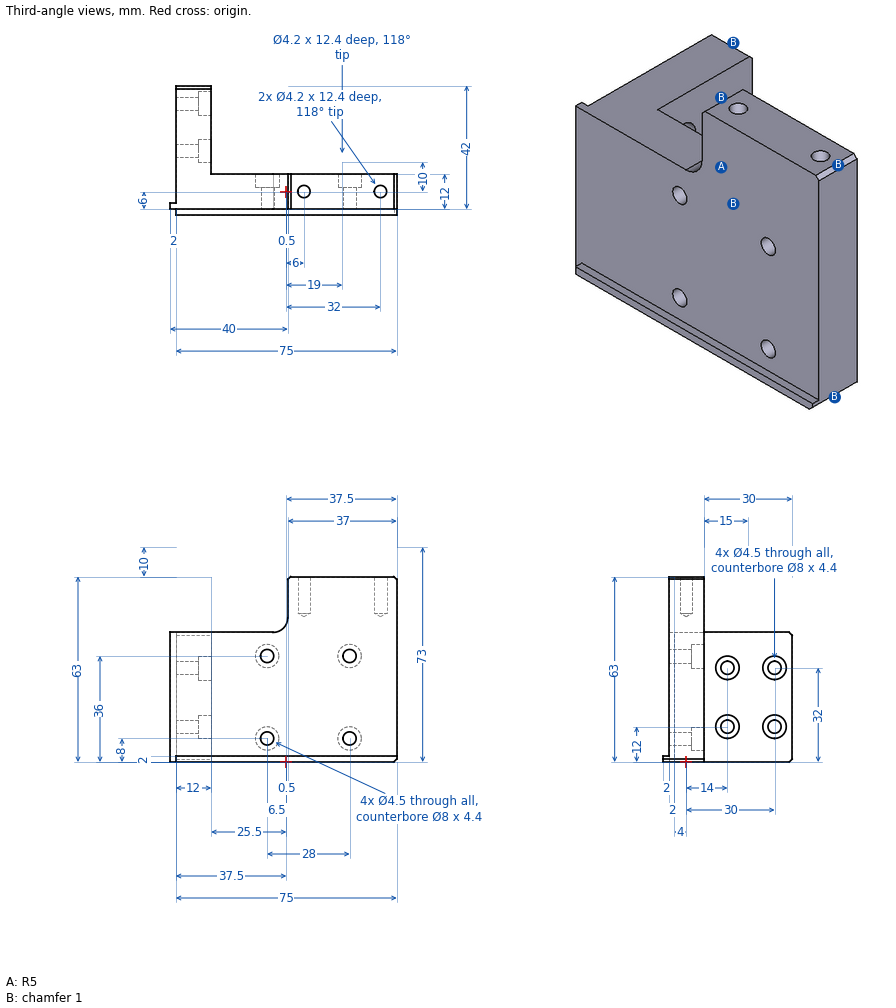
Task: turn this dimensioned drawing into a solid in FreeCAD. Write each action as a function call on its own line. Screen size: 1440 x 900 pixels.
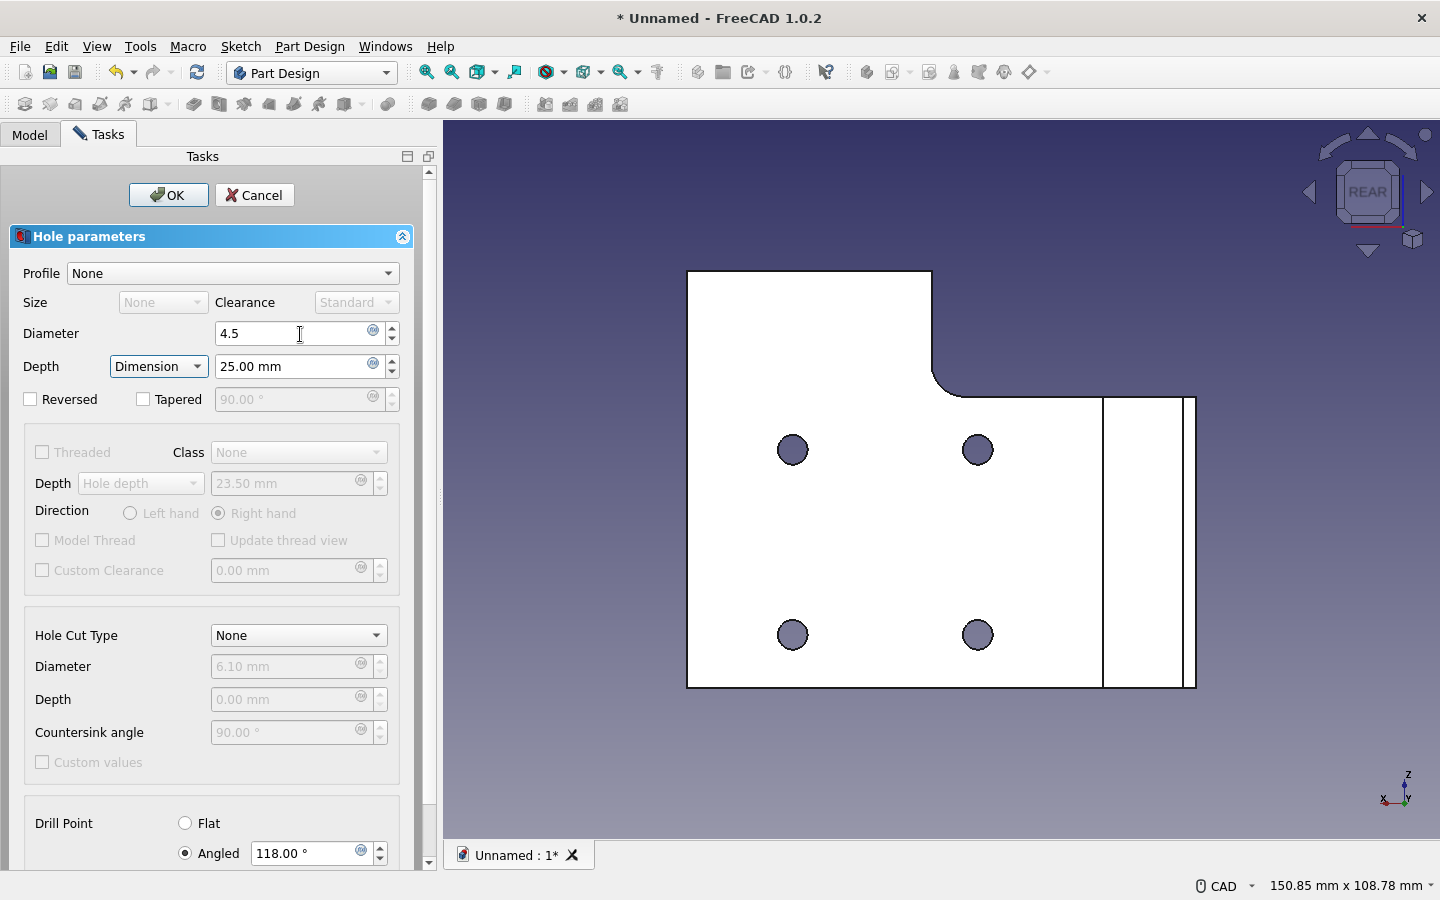
click(160, 366)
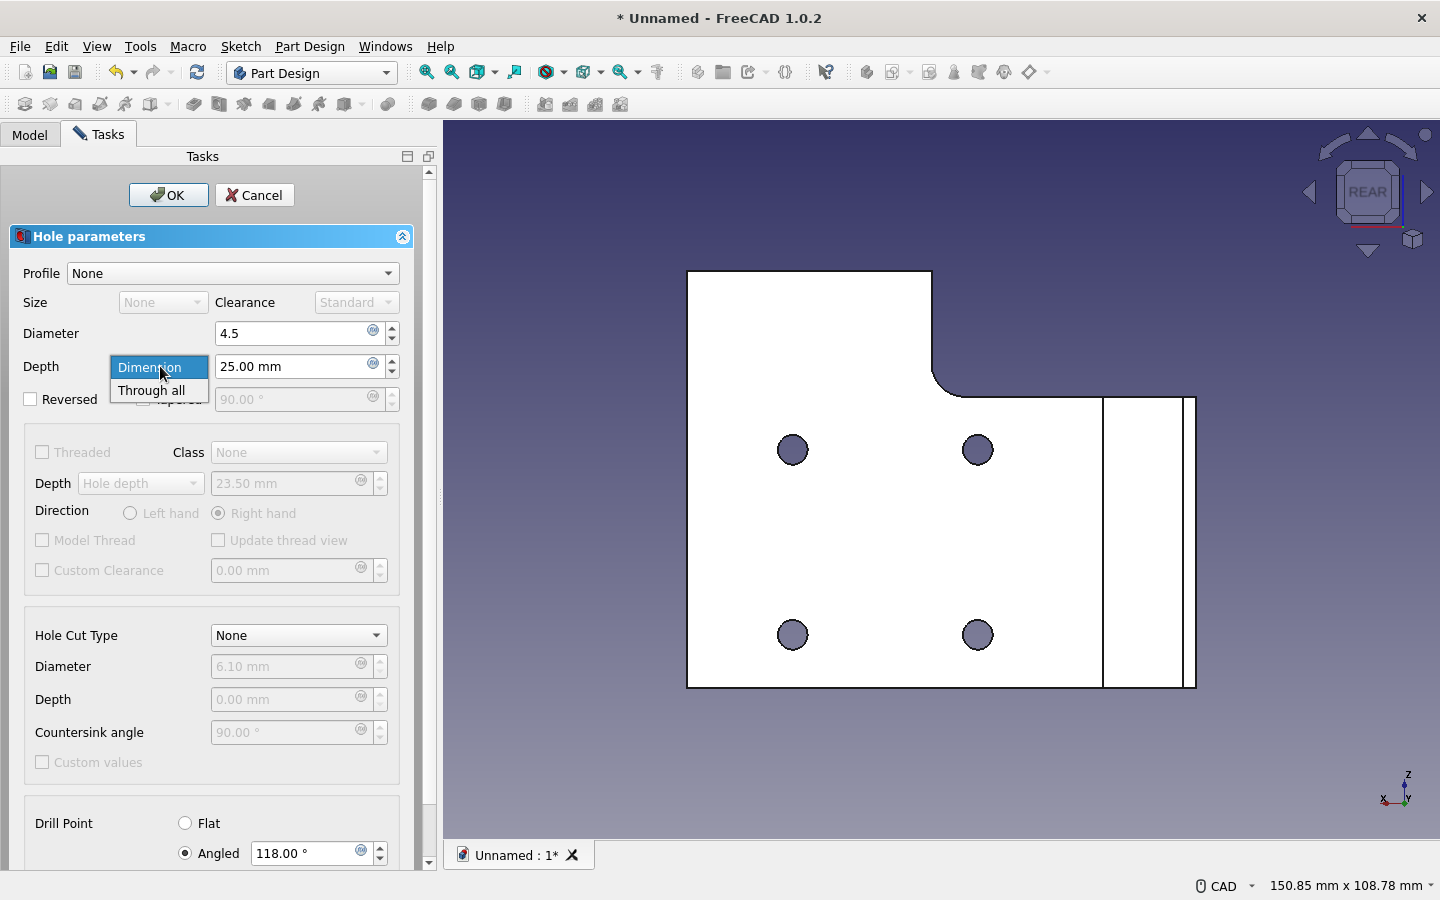
click(158, 390)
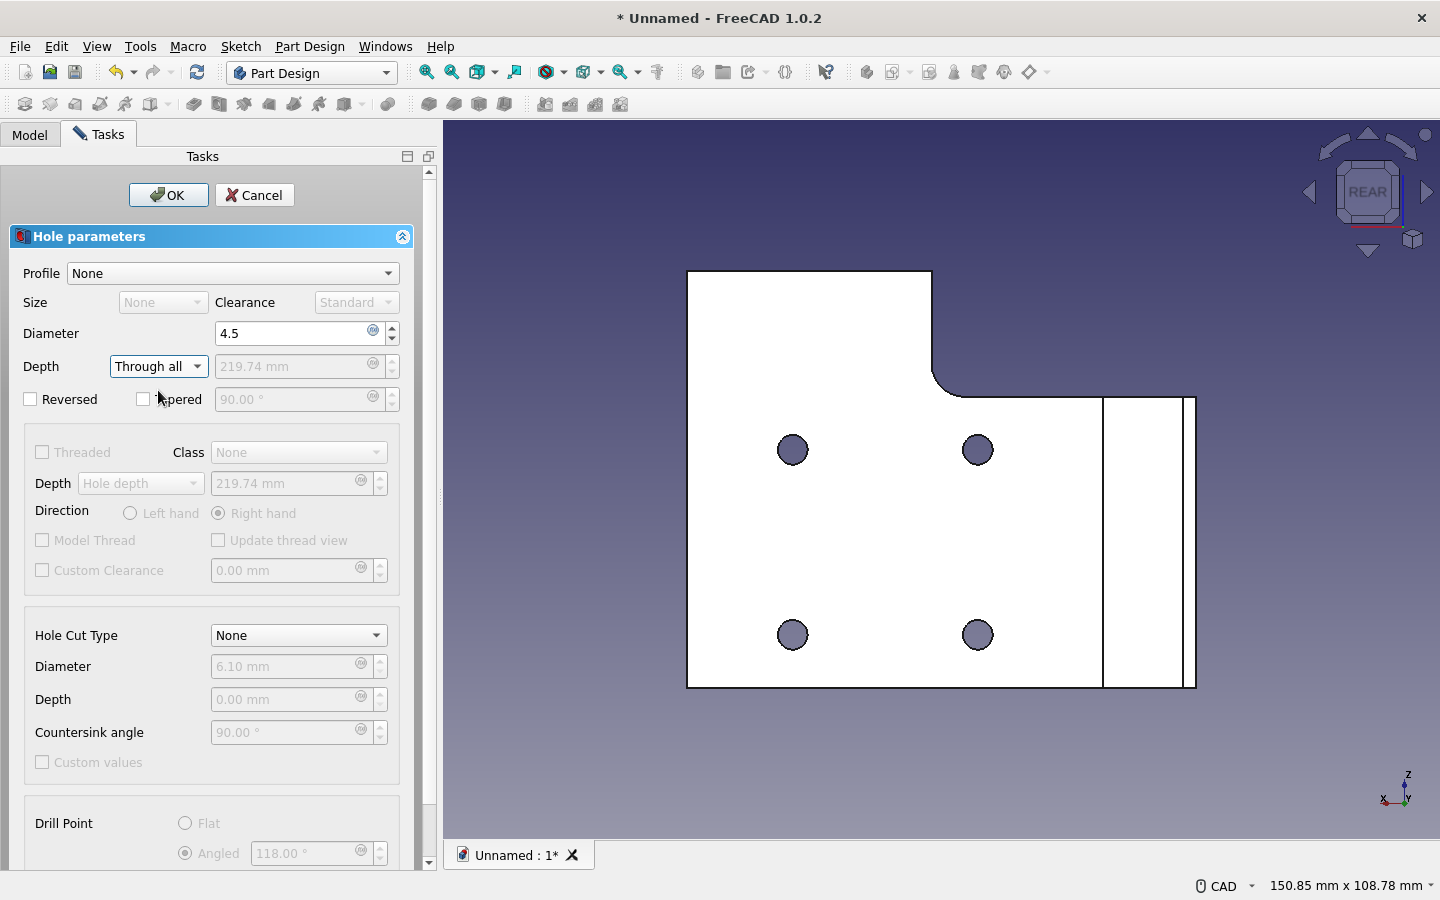
click(300, 636)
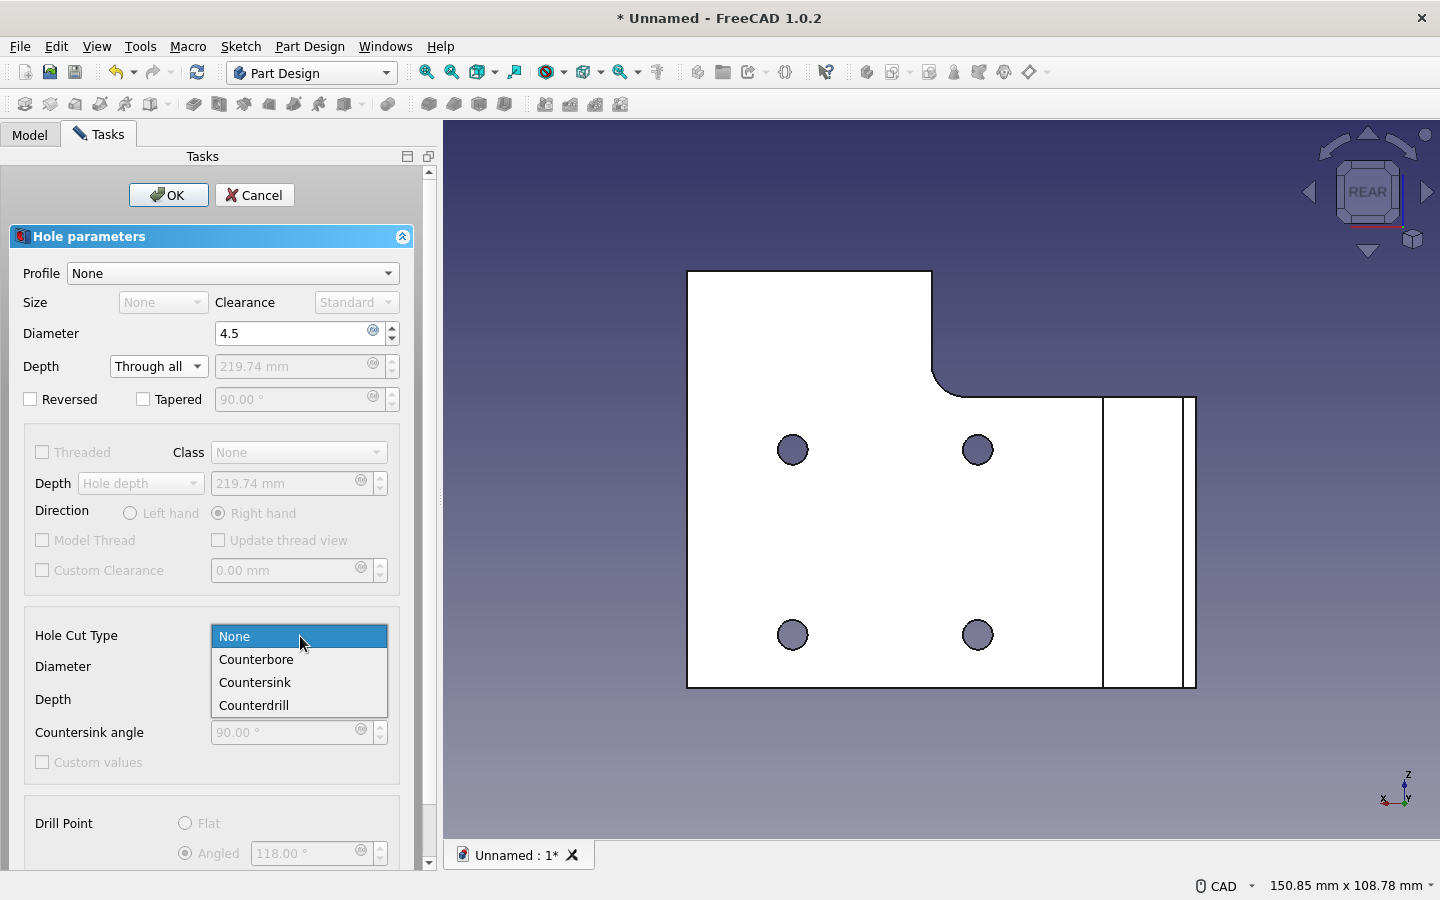
click(298, 660)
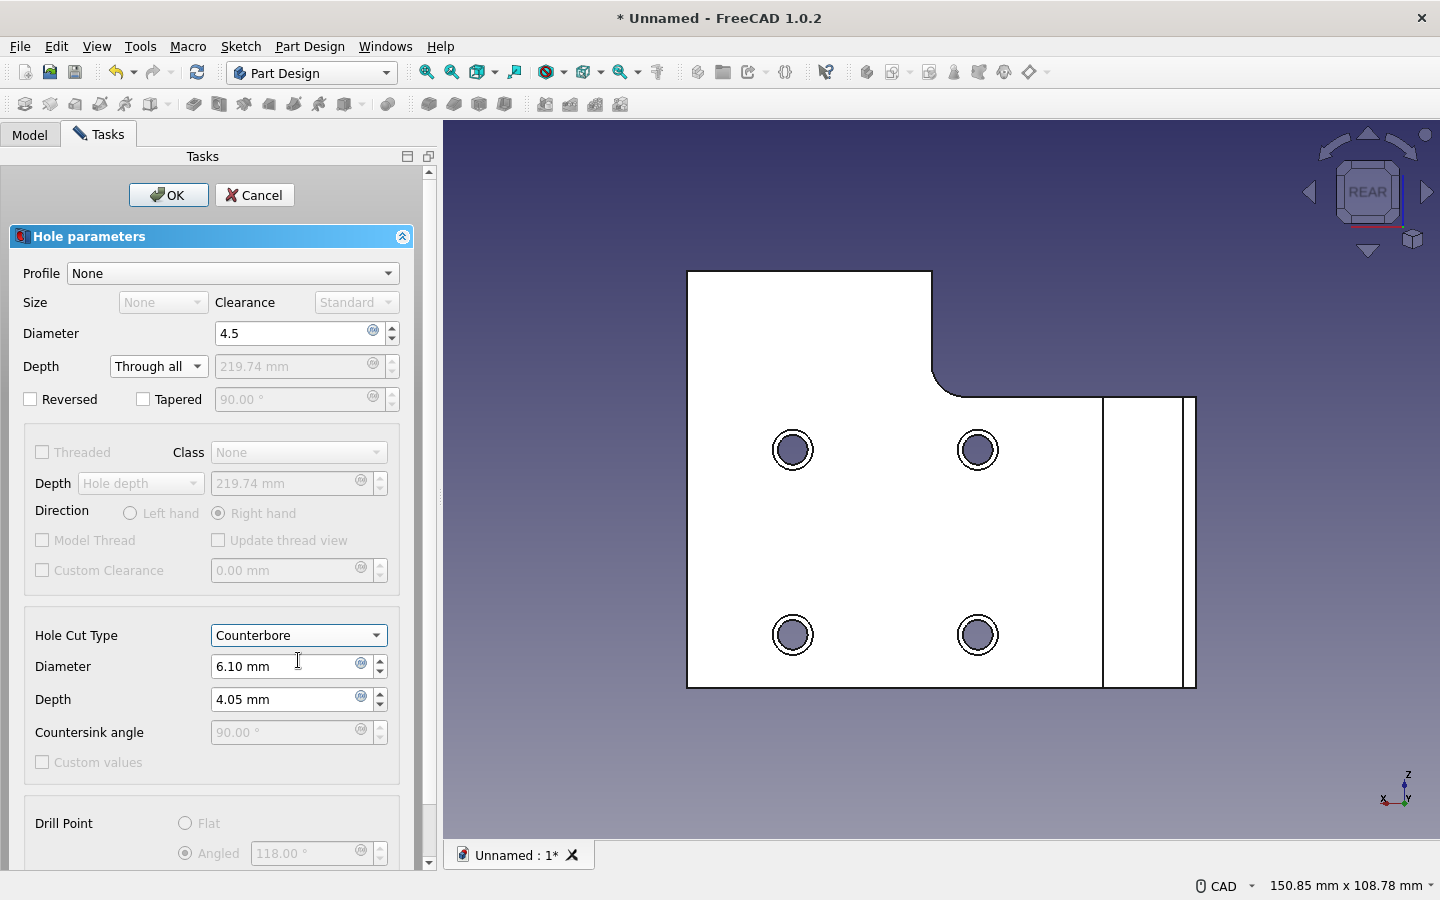
triple_click(292, 666)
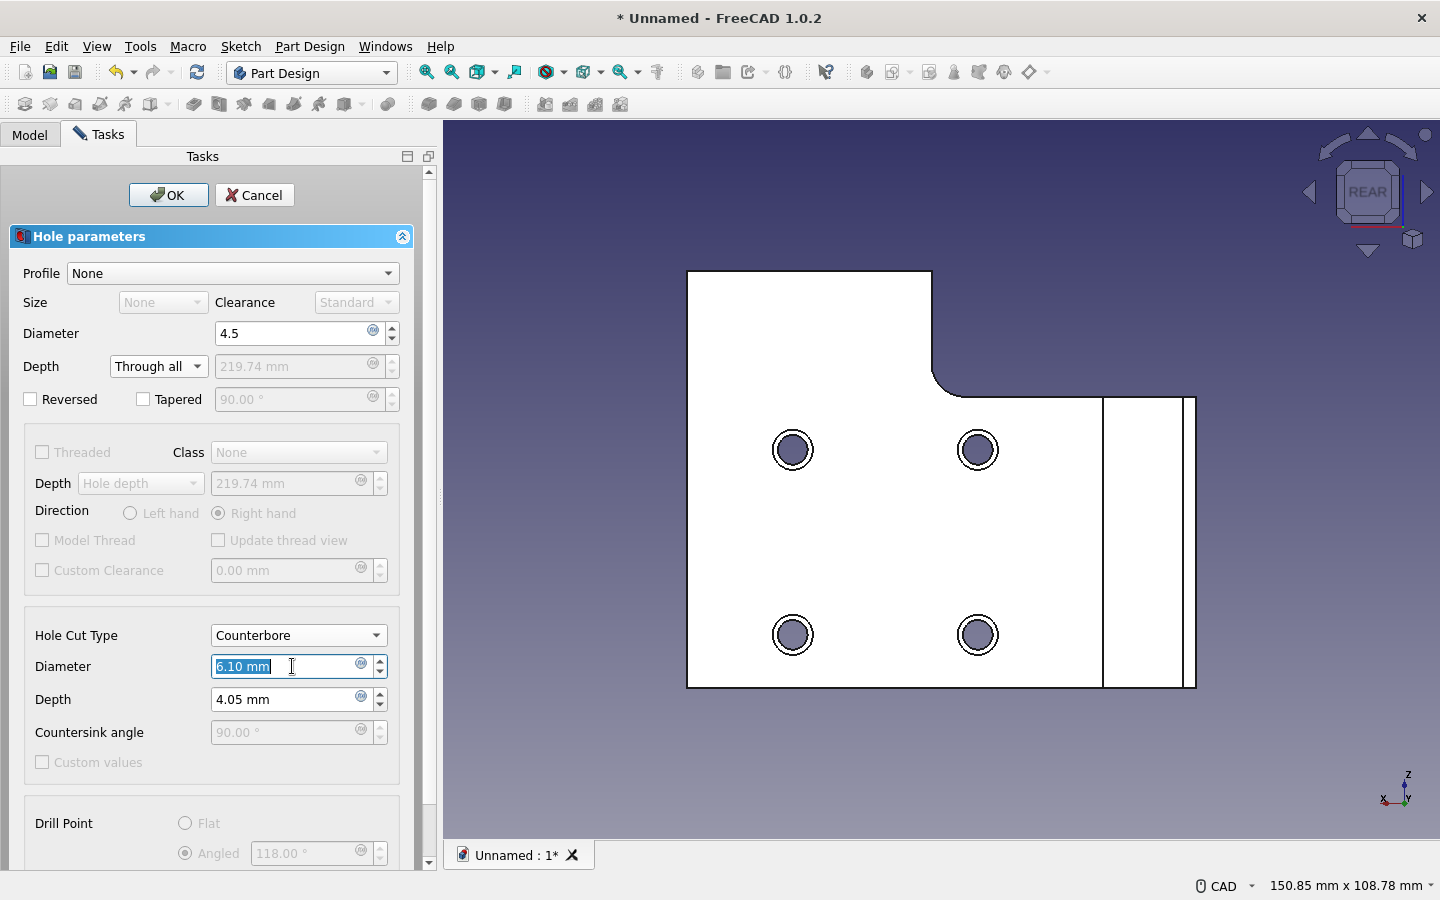
text(8)
key(Tab)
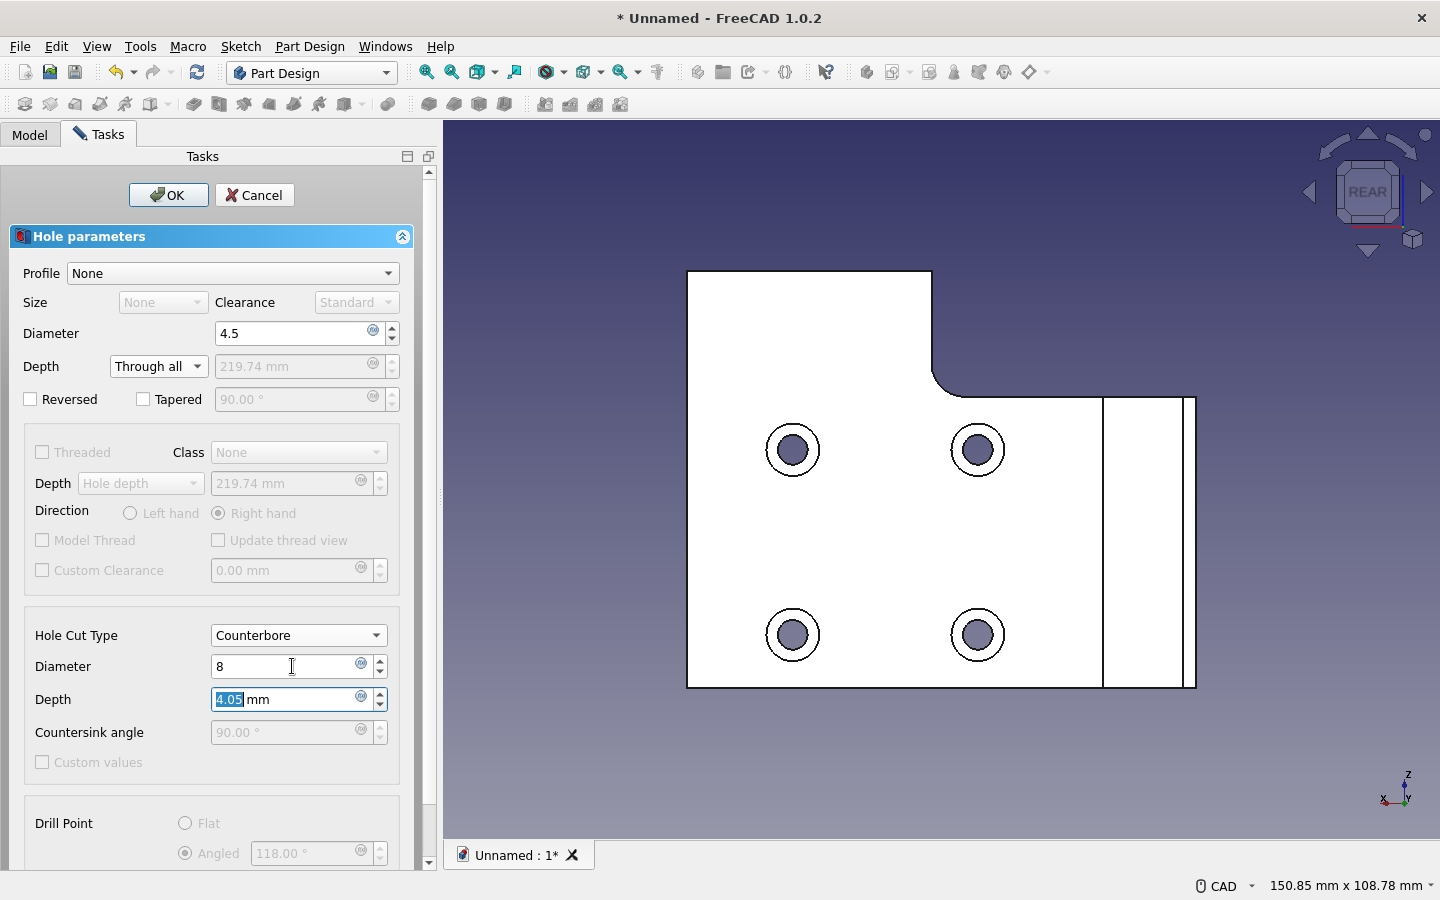
text(4.4)
key(Tab)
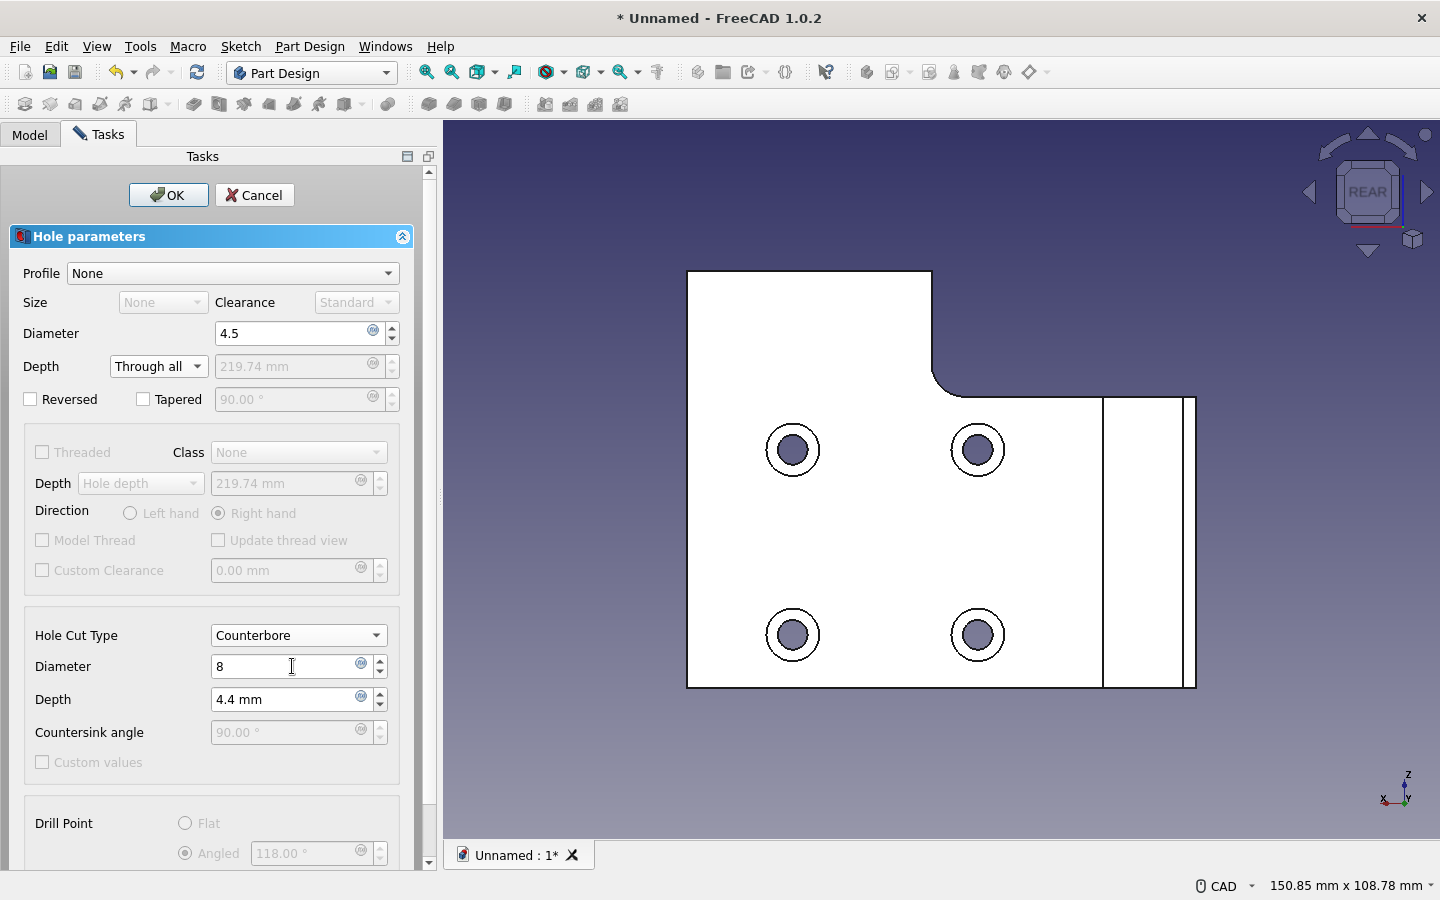
click(169, 195)